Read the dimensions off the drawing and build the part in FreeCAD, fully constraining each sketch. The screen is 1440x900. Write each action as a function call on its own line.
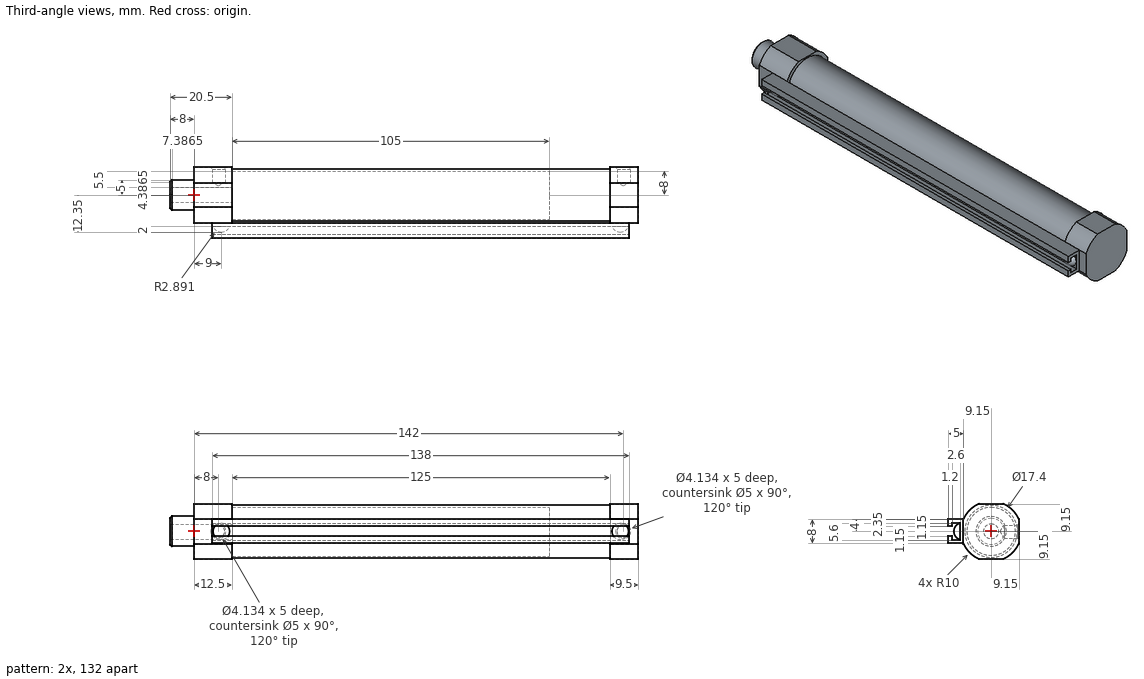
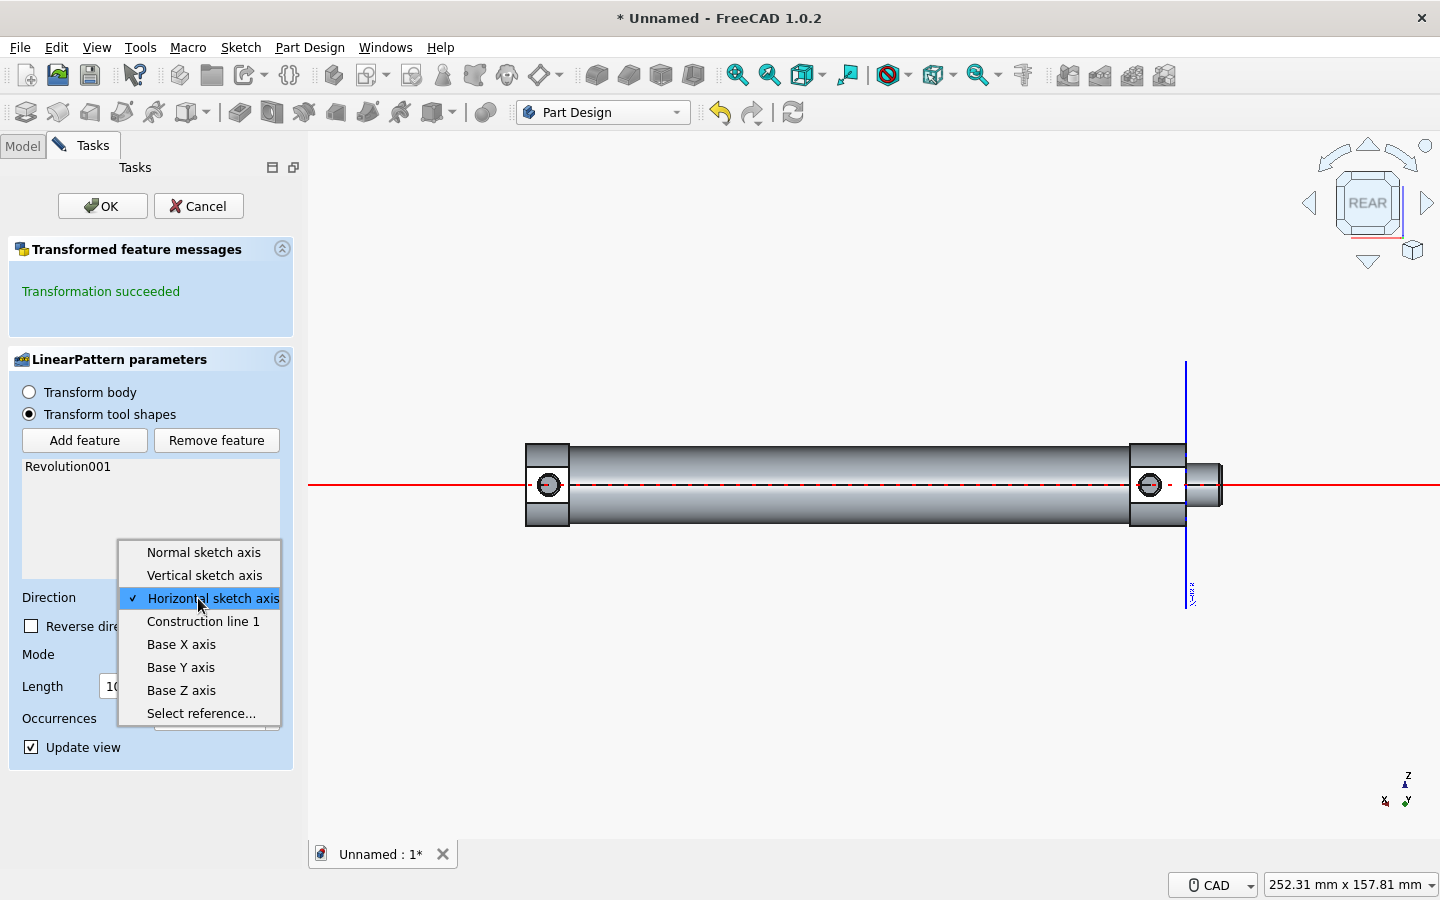
click(198, 644)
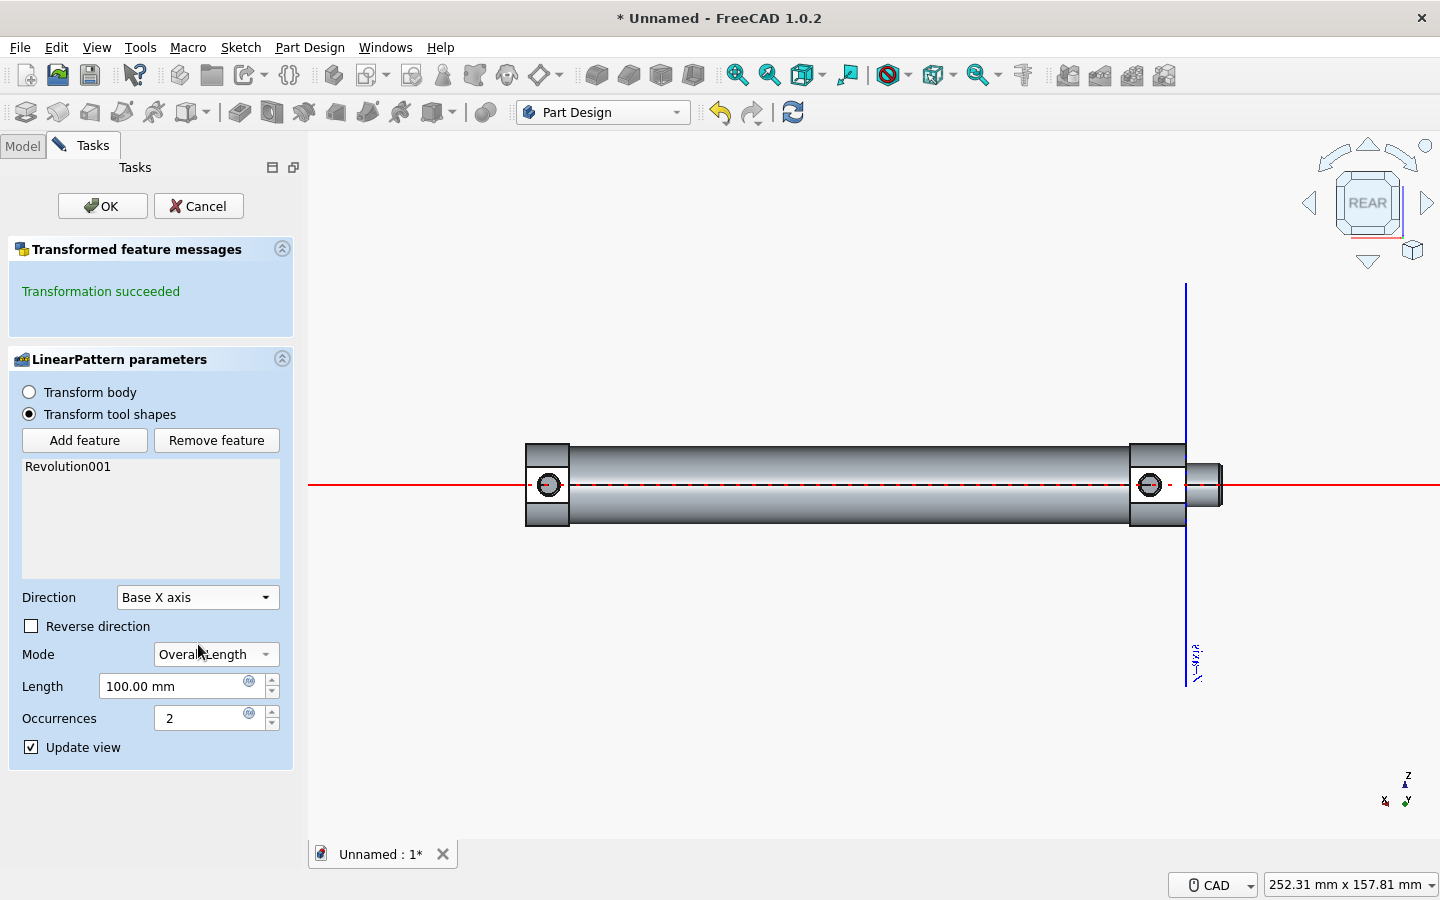
click(217, 654)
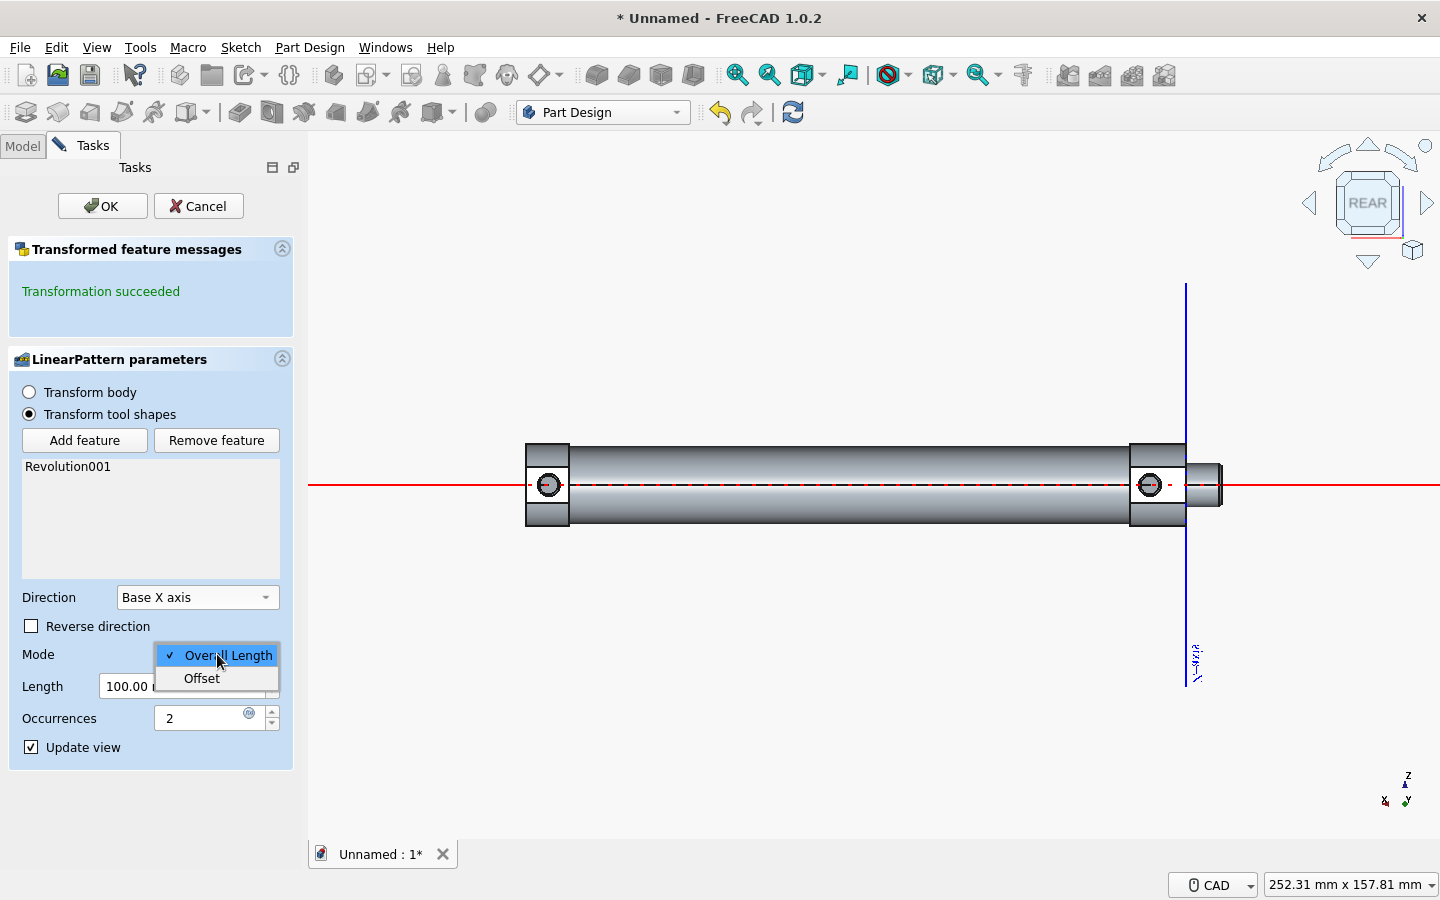
click(216, 678)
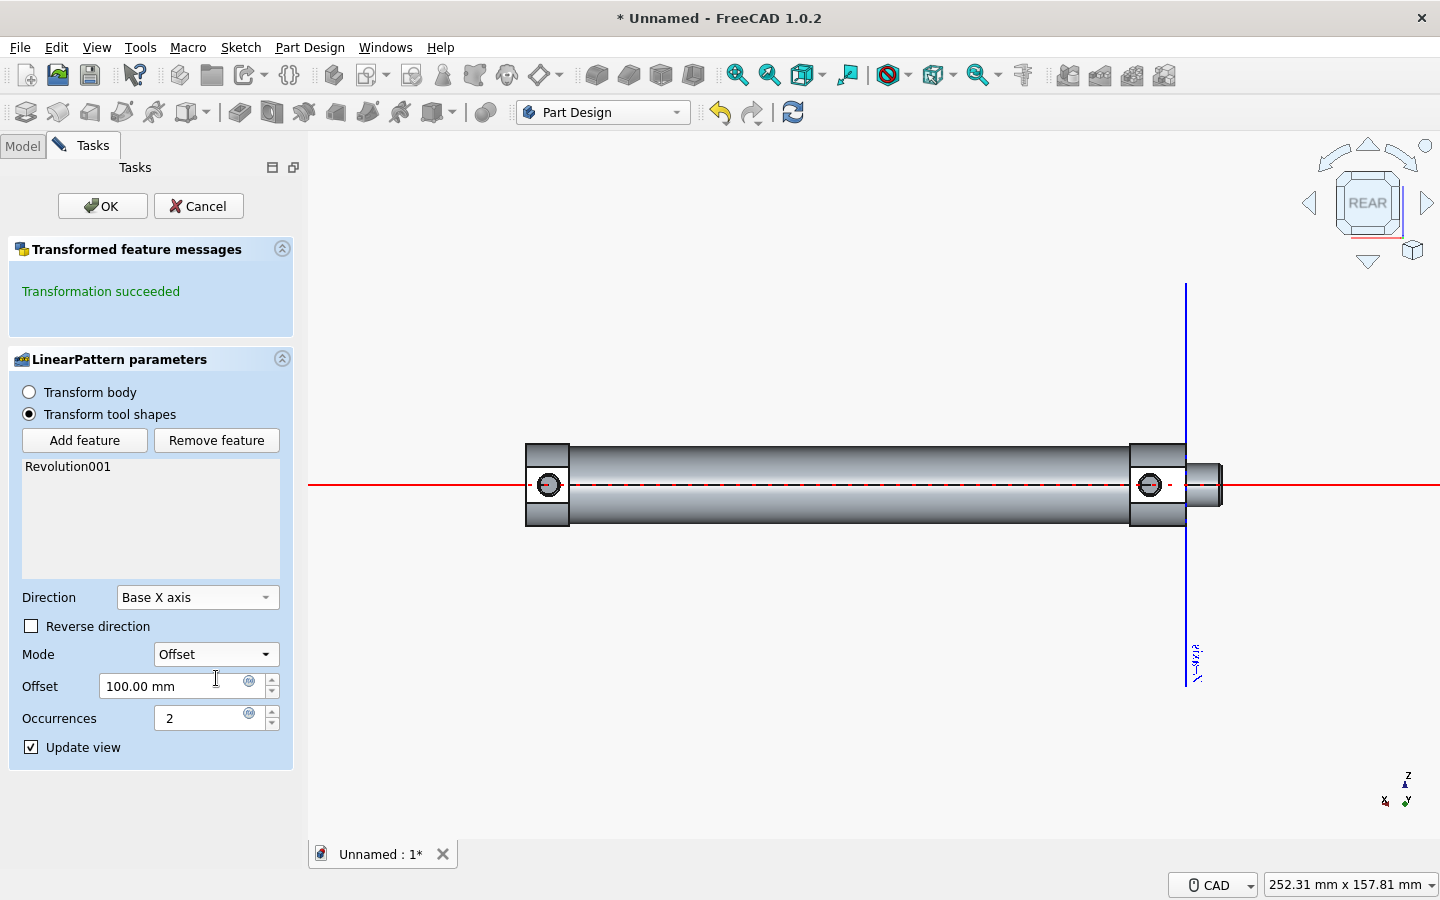
triple_click(182, 686)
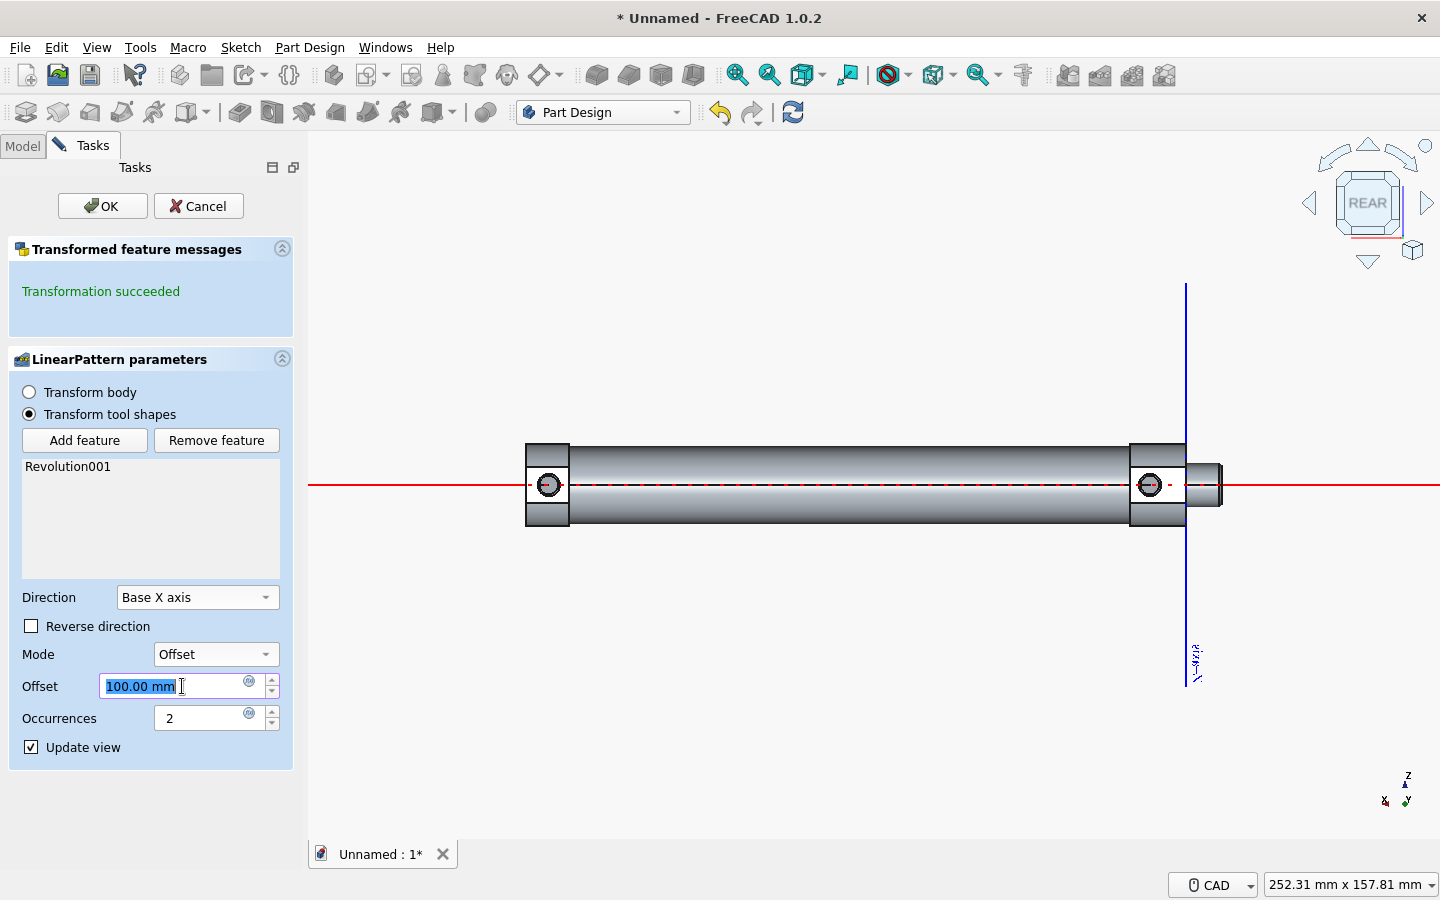
text(132)
key(Tab)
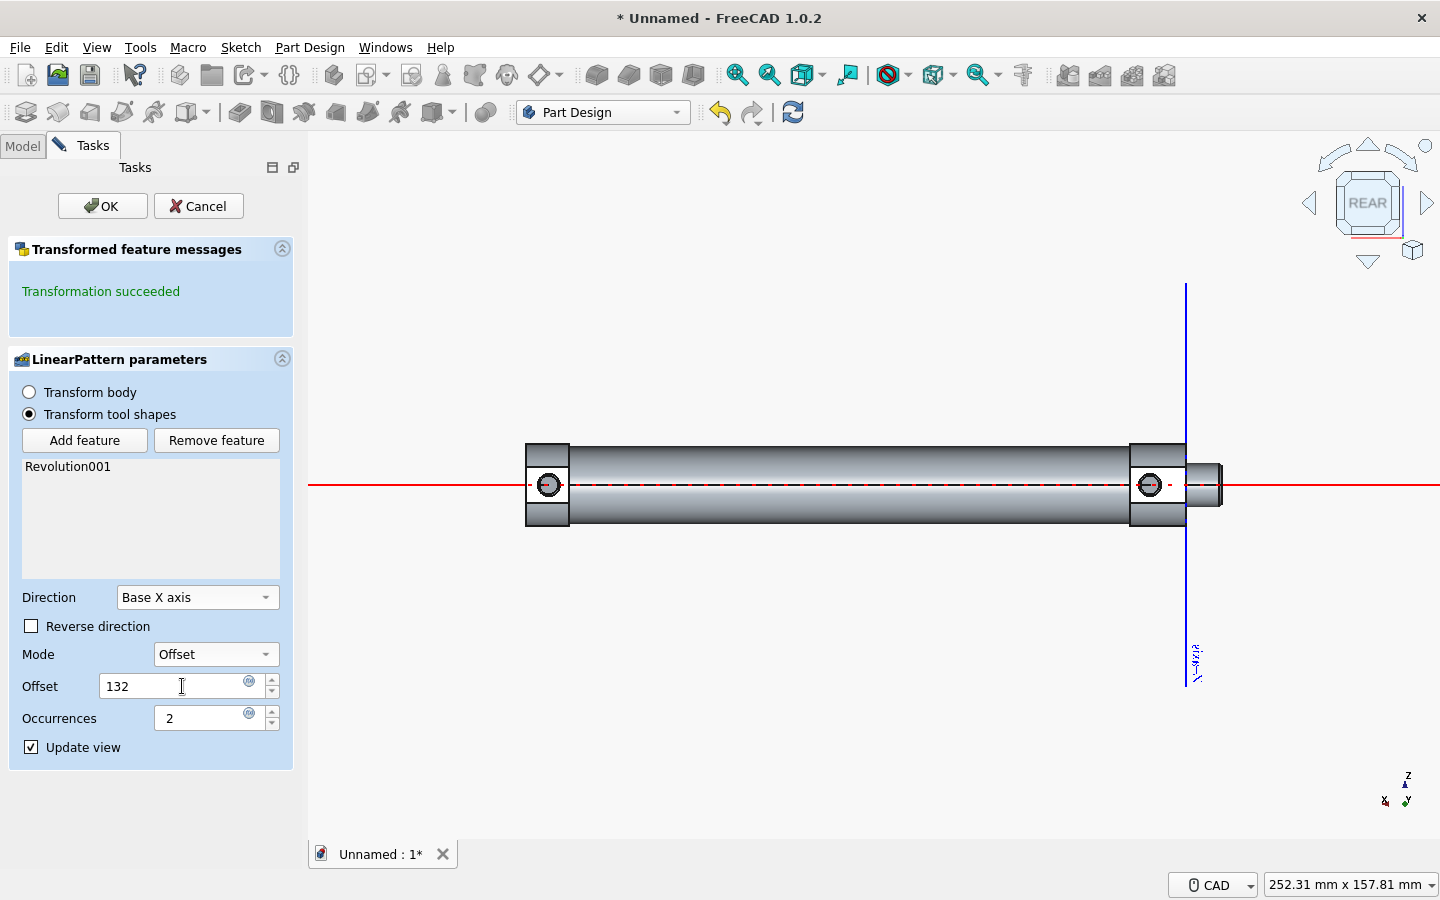
triple_click(209, 718)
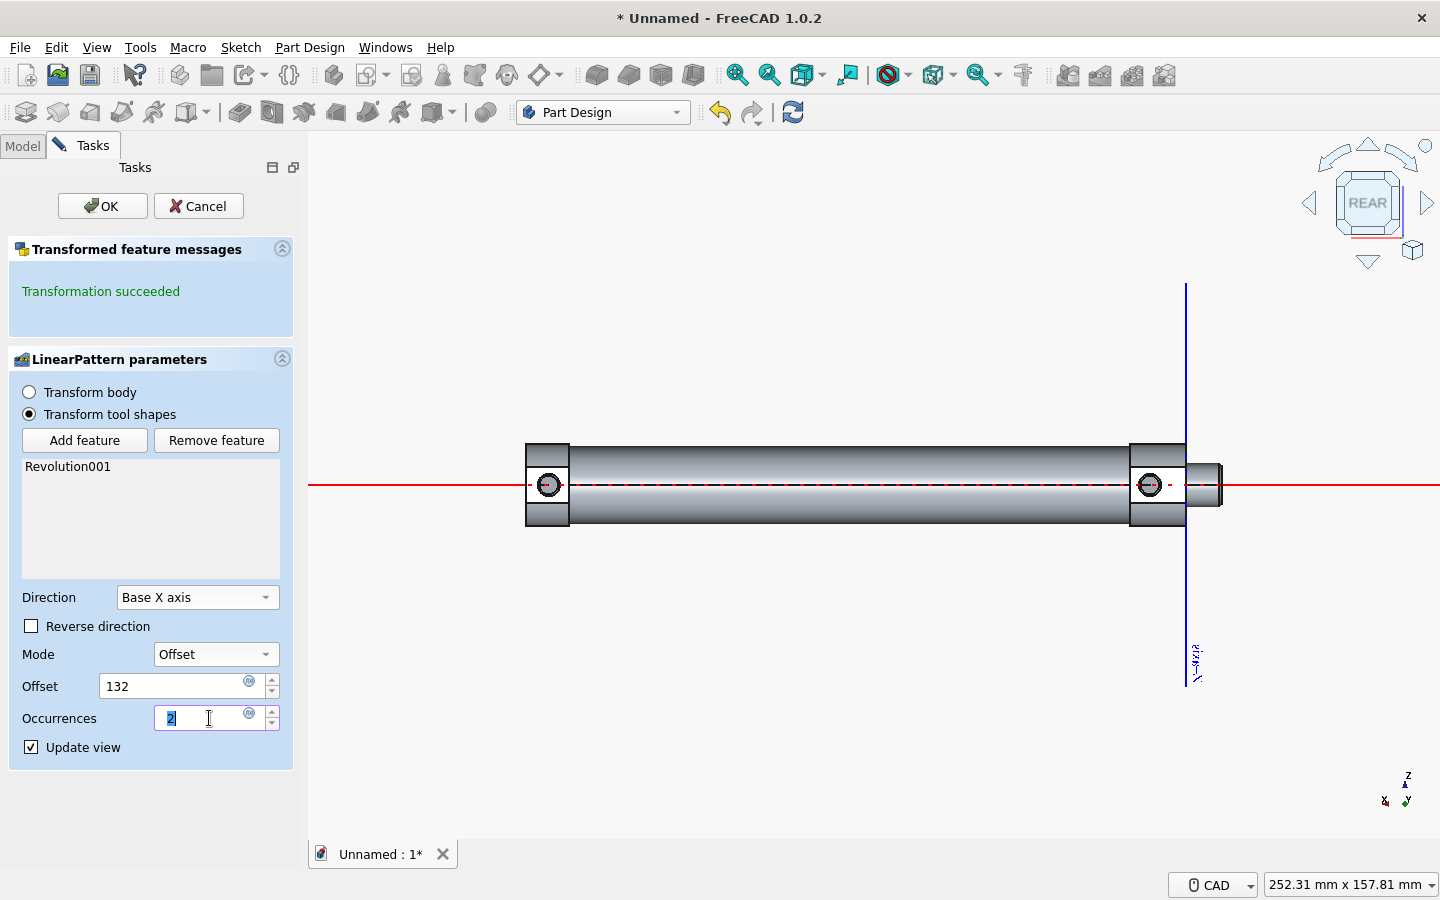
text(2)
key(Tab)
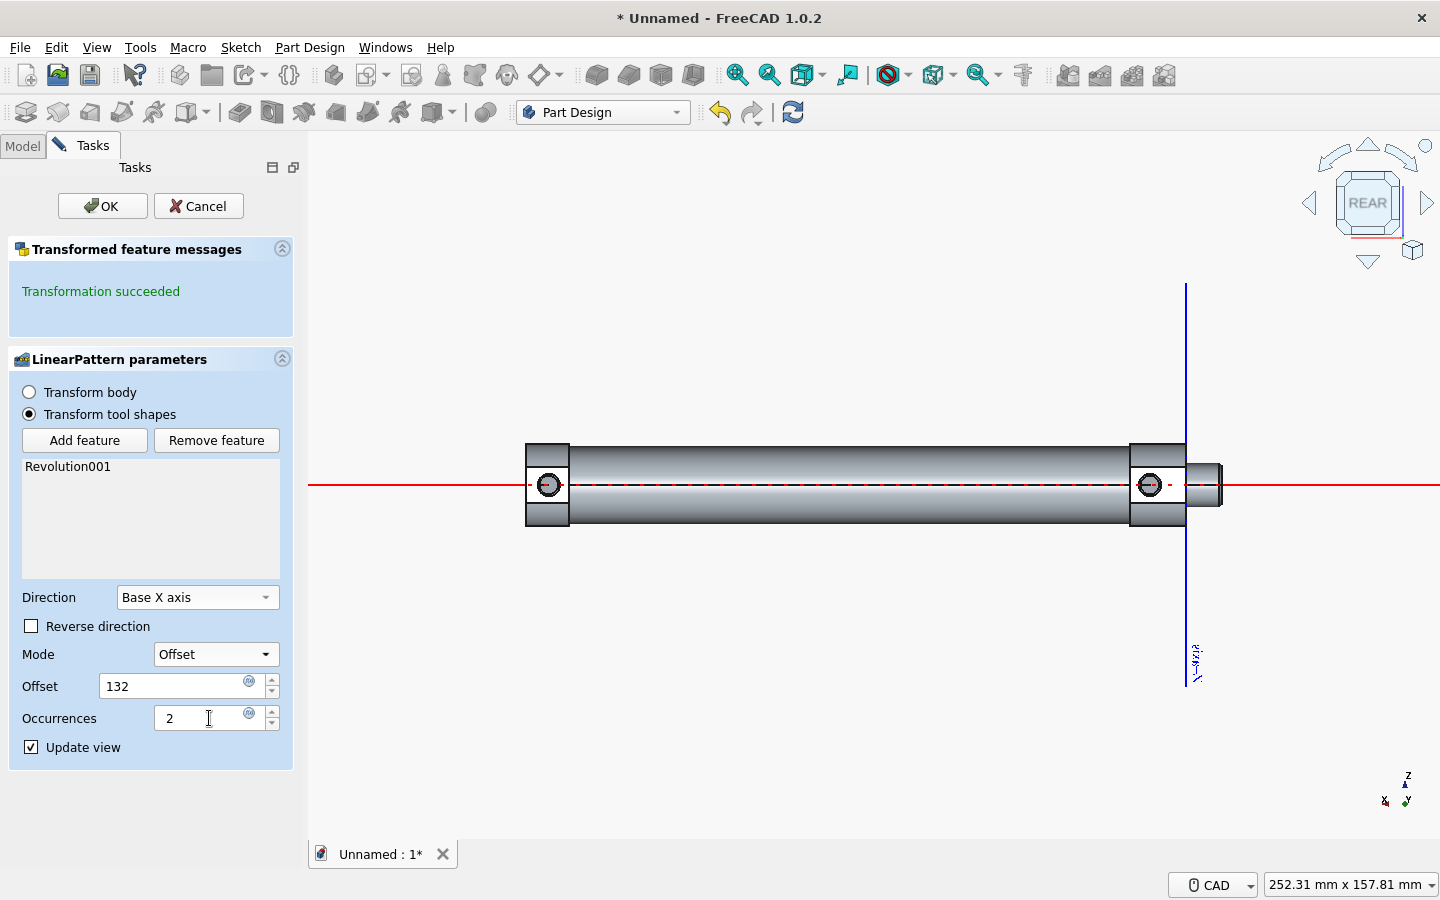
click(103, 206)